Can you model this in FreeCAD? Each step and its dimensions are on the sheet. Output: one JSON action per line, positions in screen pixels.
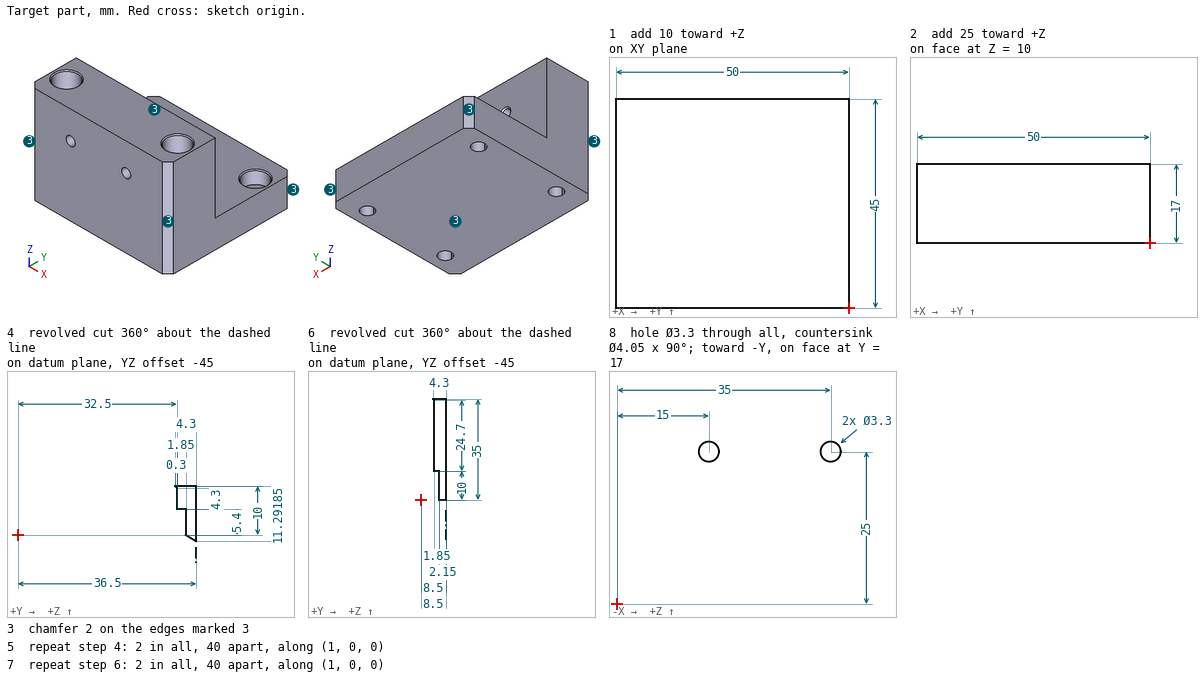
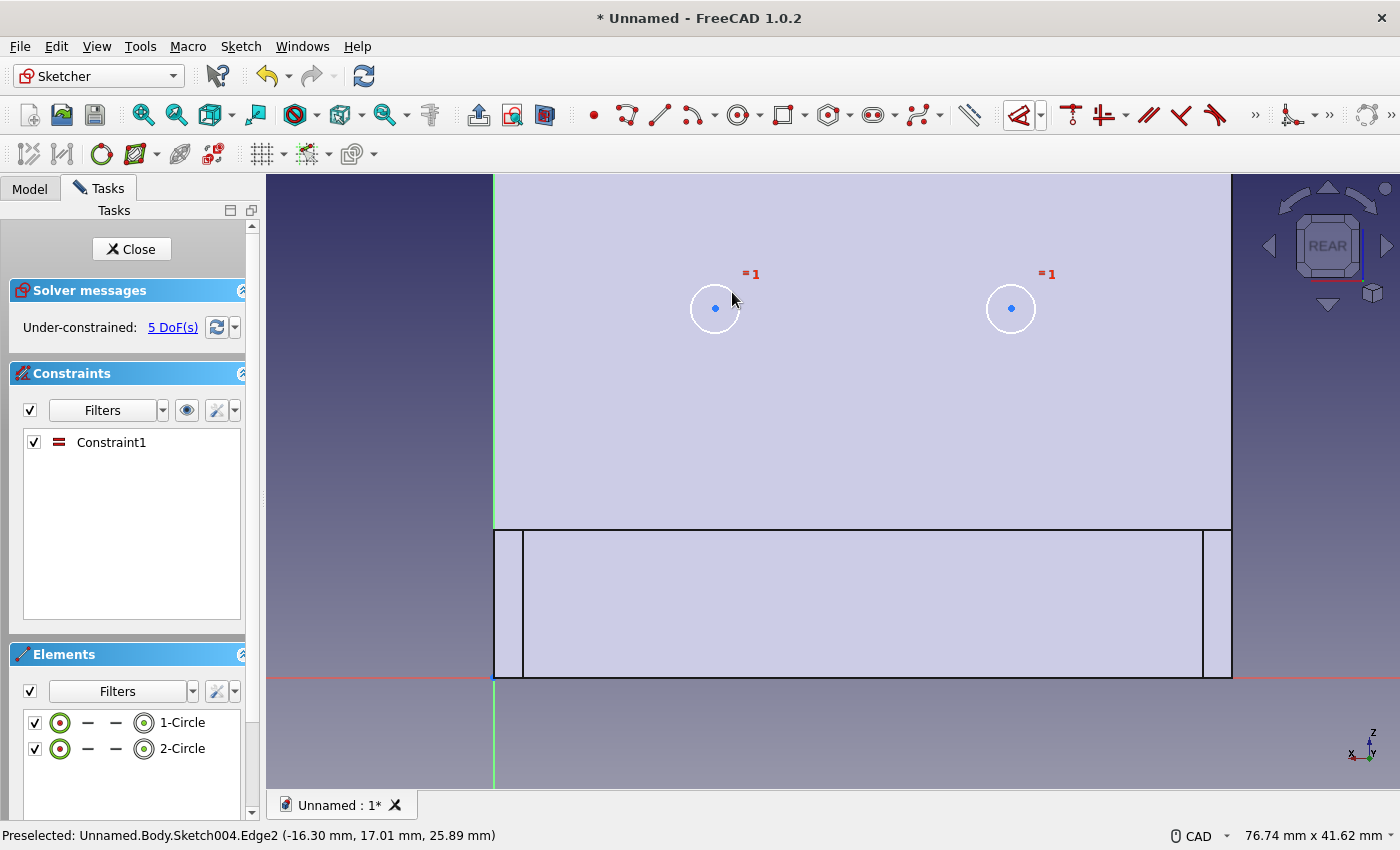
{"action": "left_click", "coordinate": [1011, 309]}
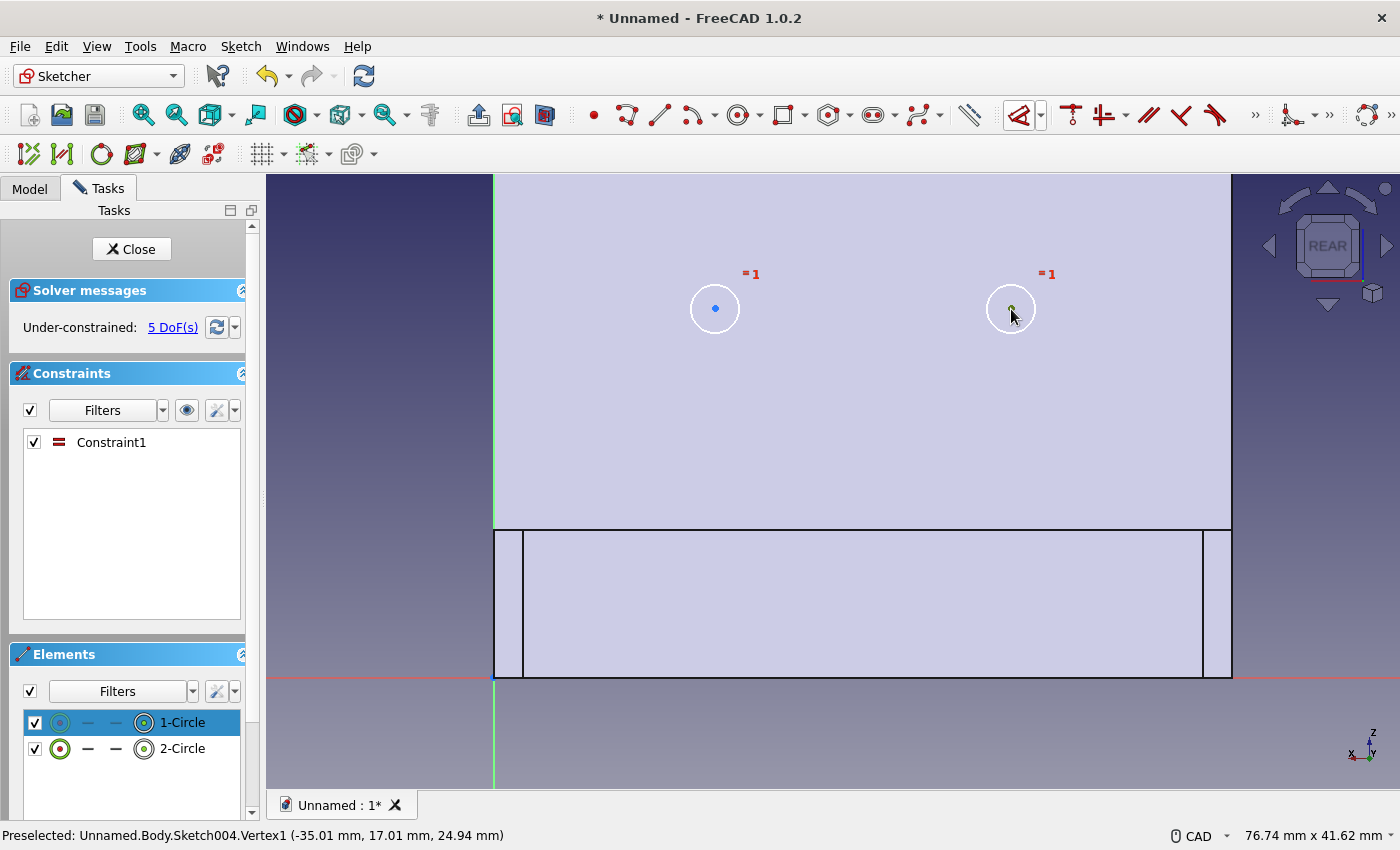
{"action": "left_click", "coordinate": [715, 309]}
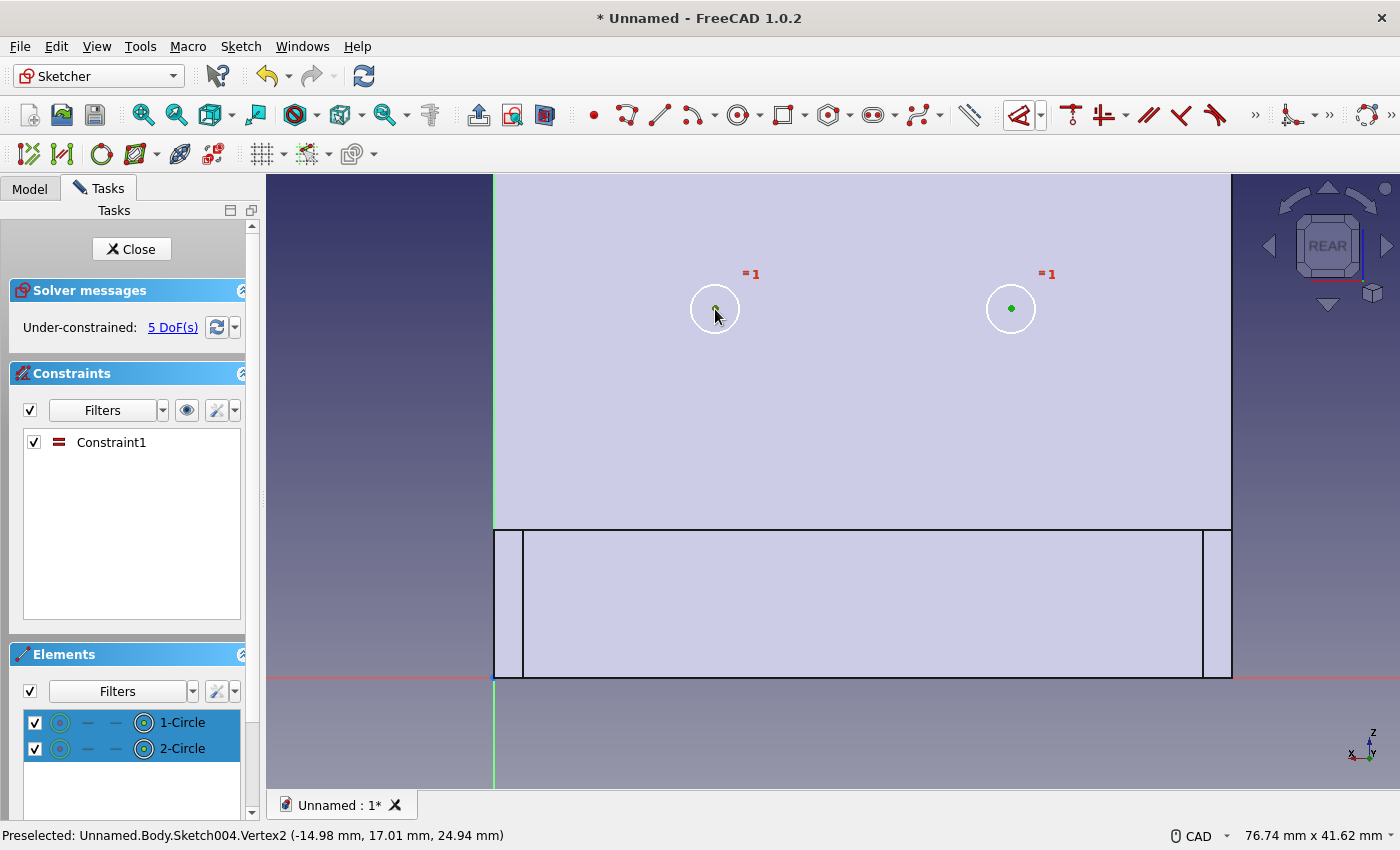
{"action": "left_click", "coordinate": [1126, 116]}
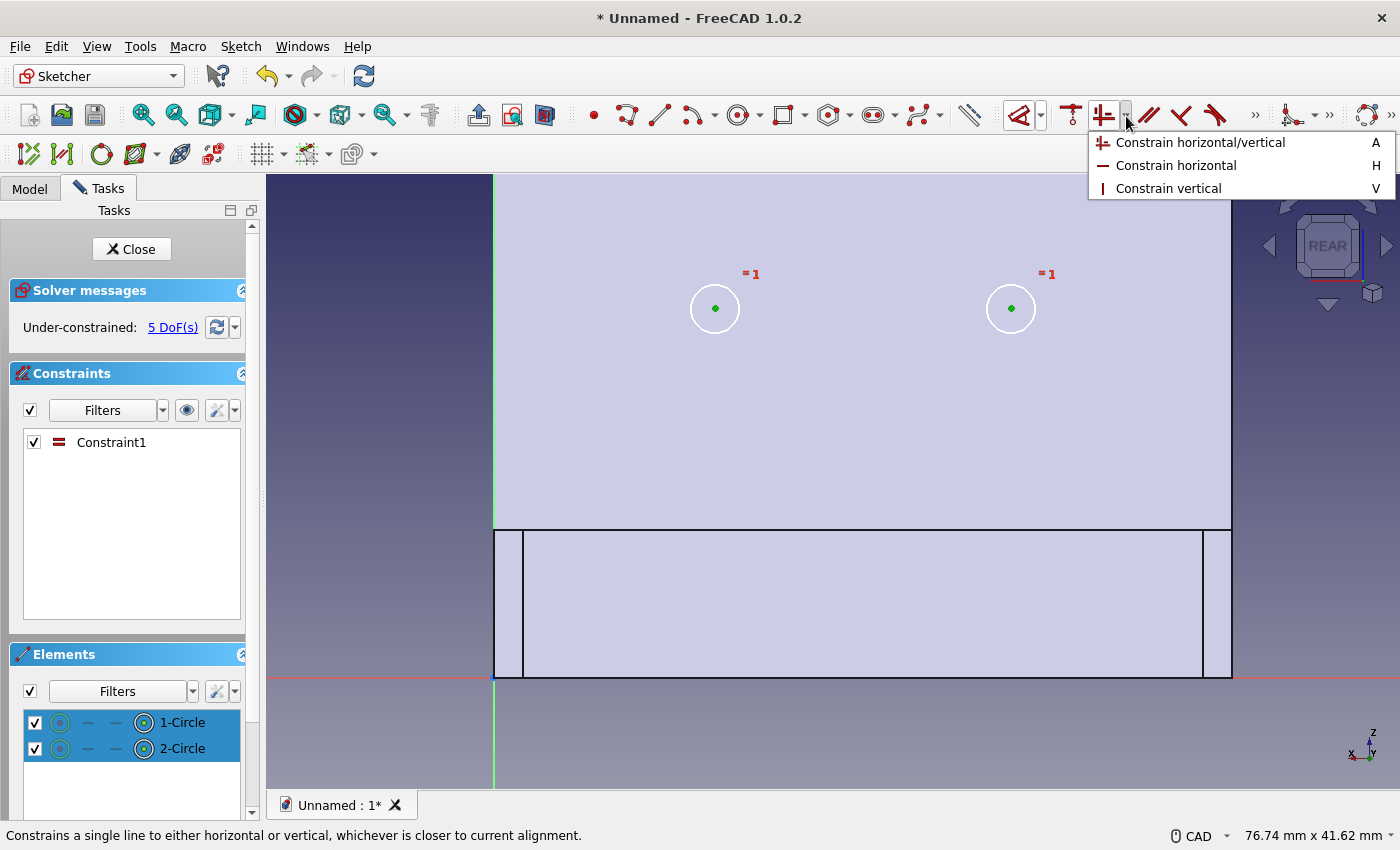
{"action": "left_click", "coordinate": [1242, 166]}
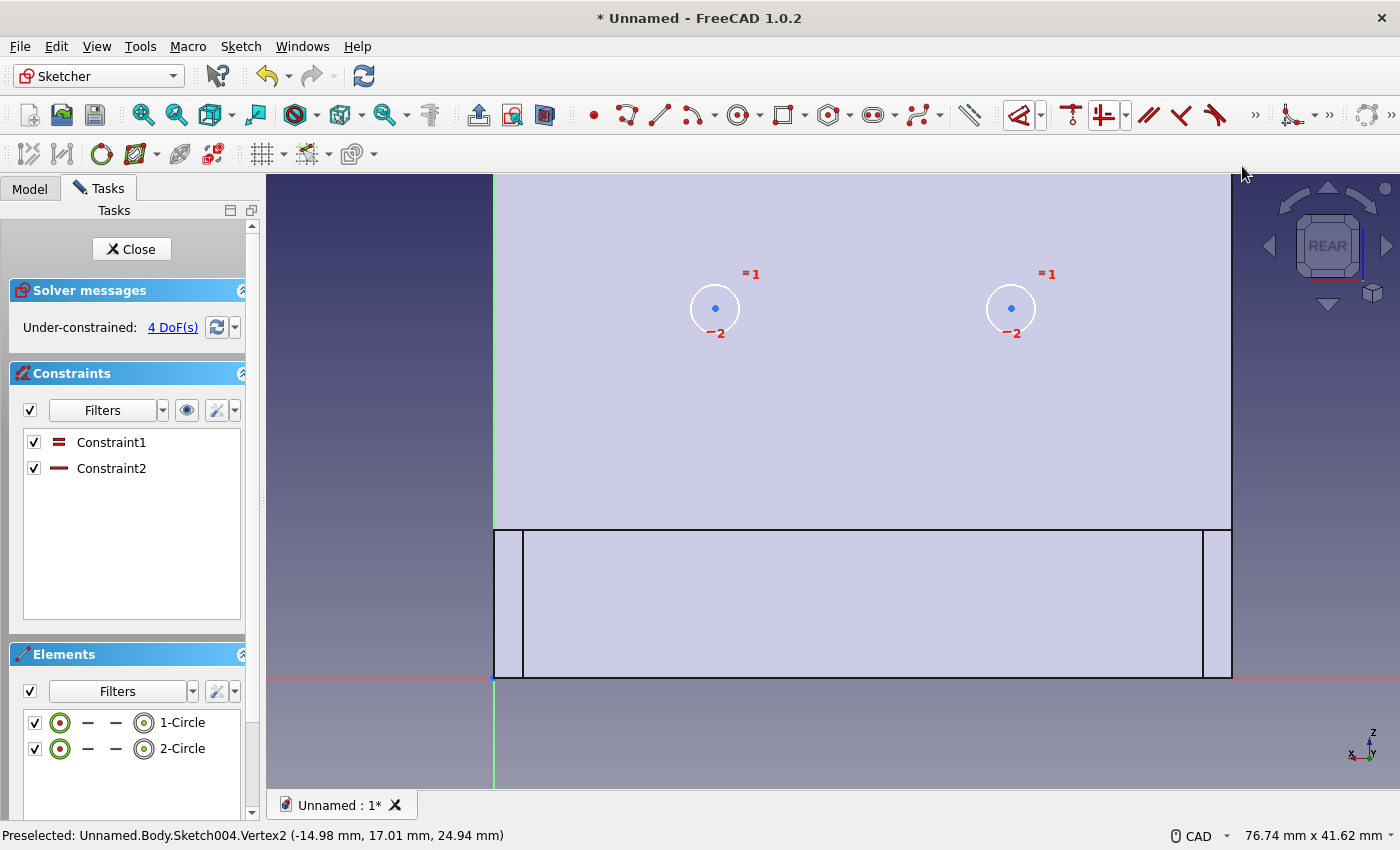
{"action": "left_click", "coordinate": [1028, 292]}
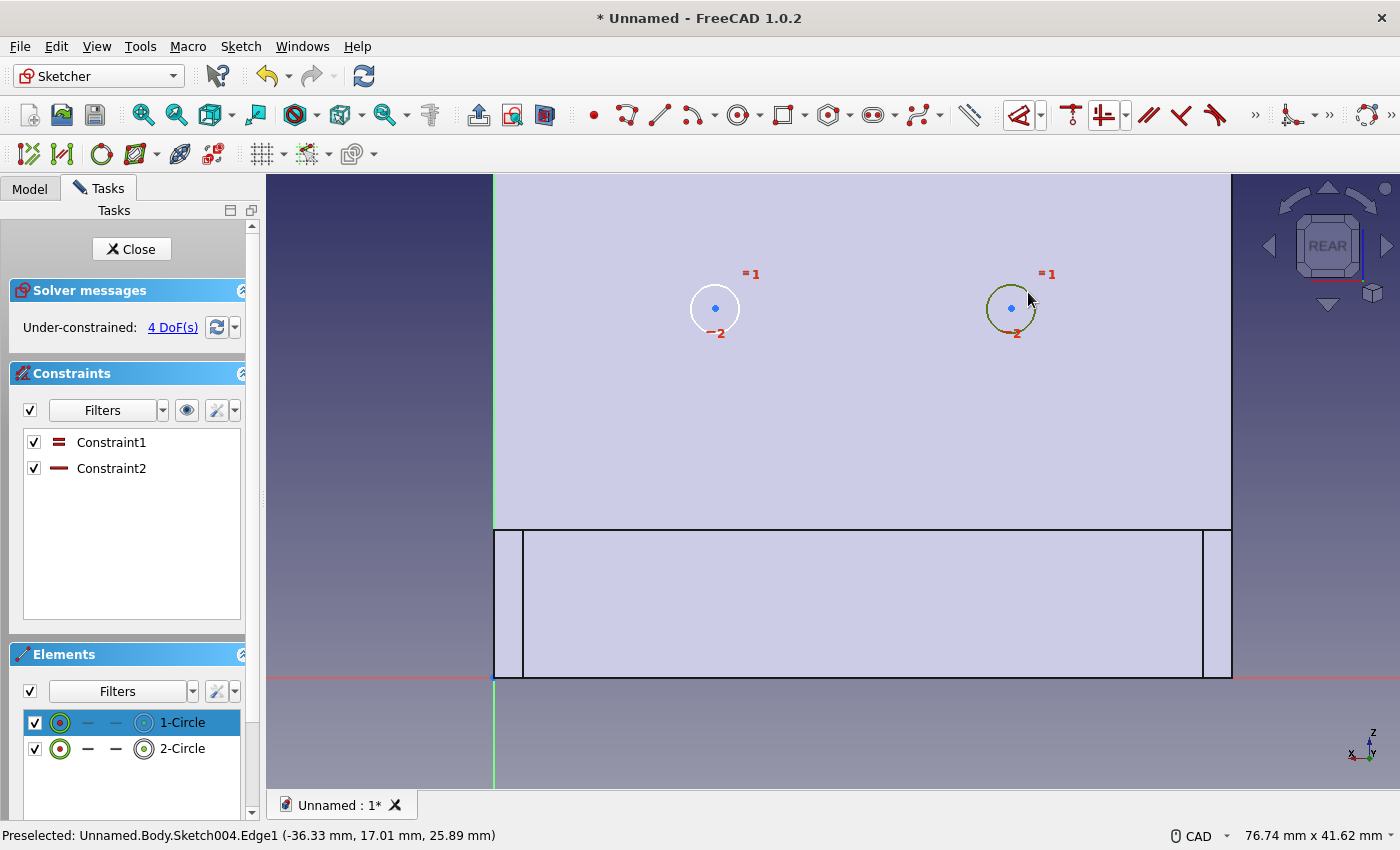
{"action": "key", "text": "k o"}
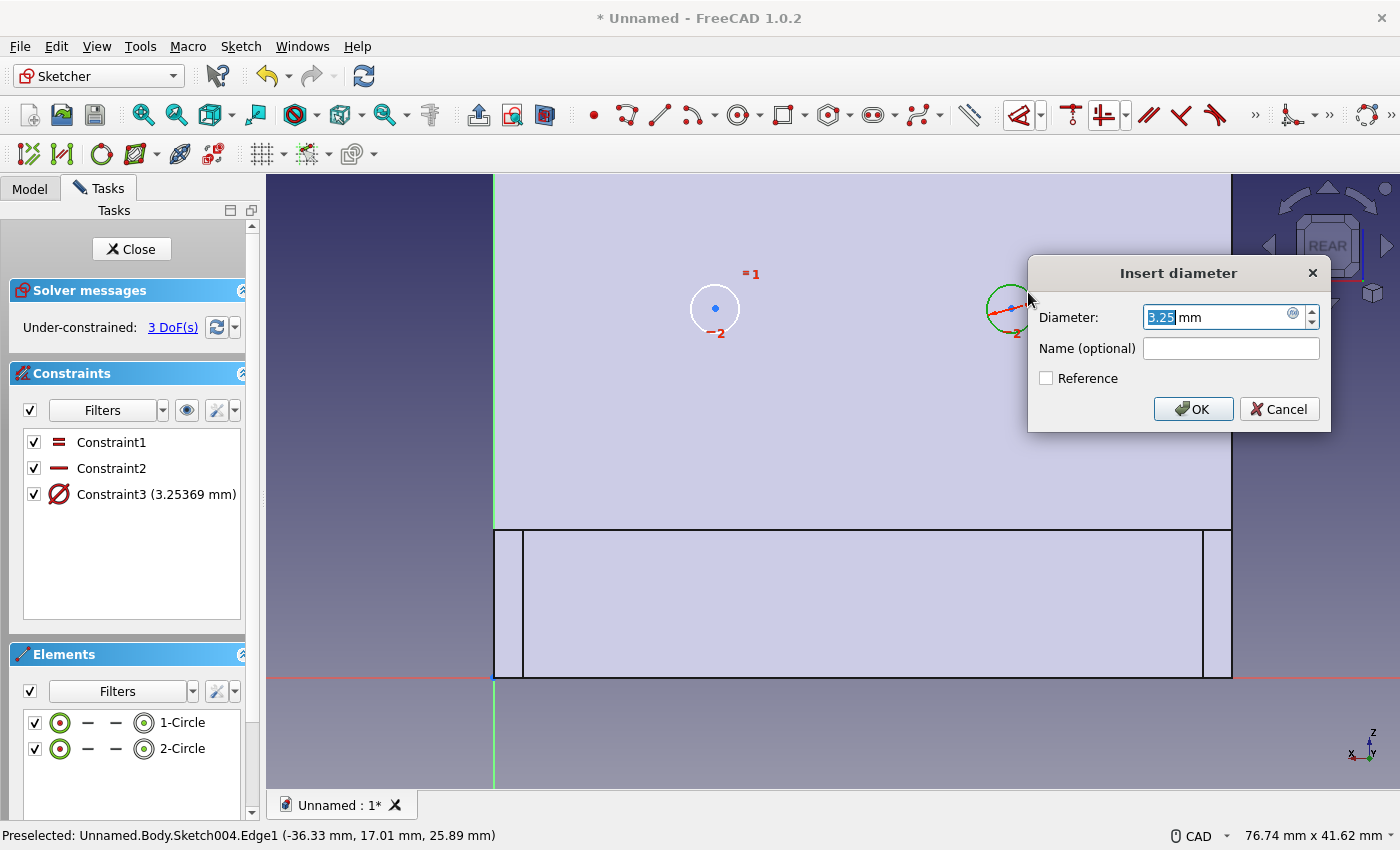
{"action": "type", "text": "3.3"}
{"action": "key", "text": "Return"}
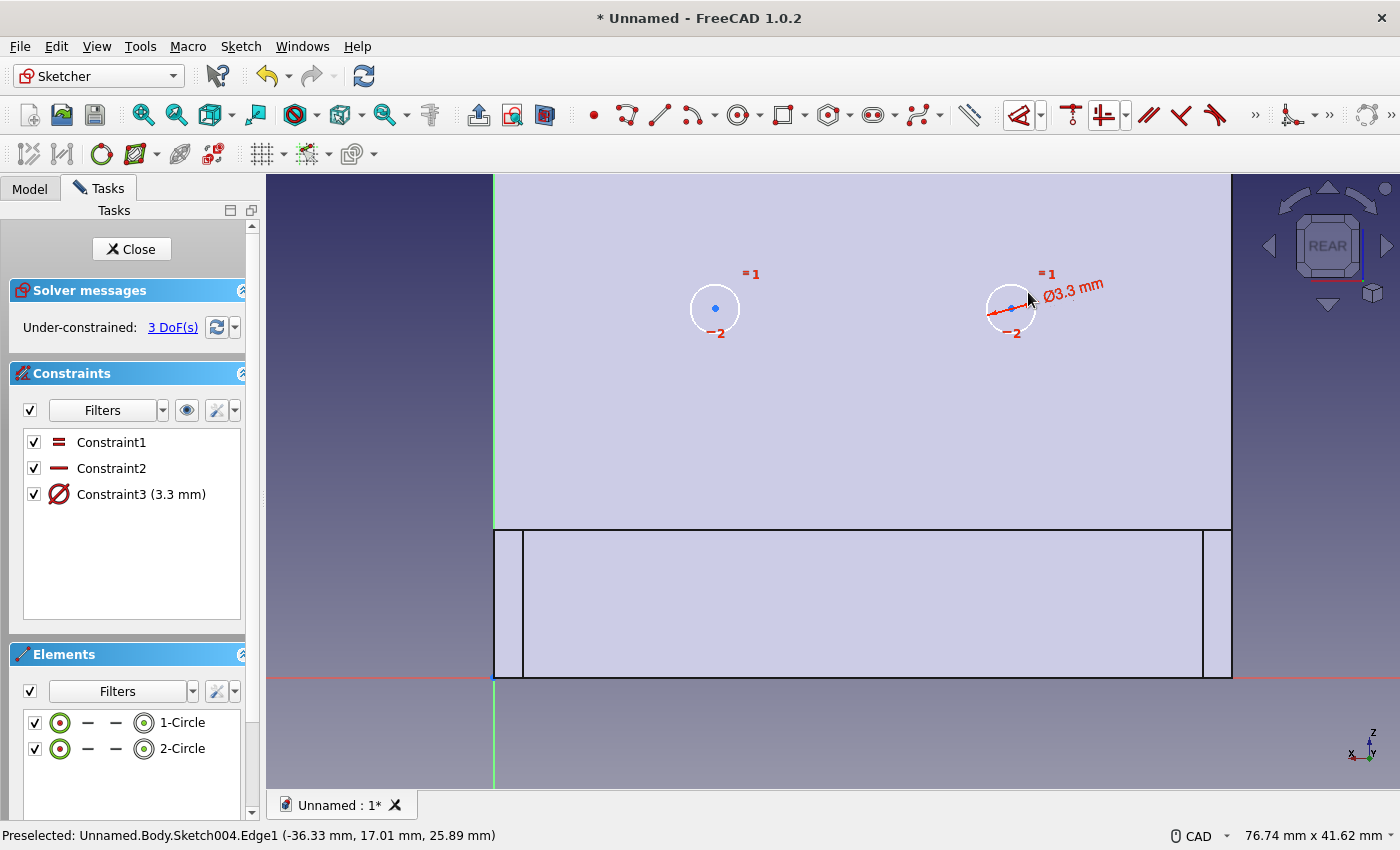
{"action": "left_click", "coordinate": [1011, 309]}